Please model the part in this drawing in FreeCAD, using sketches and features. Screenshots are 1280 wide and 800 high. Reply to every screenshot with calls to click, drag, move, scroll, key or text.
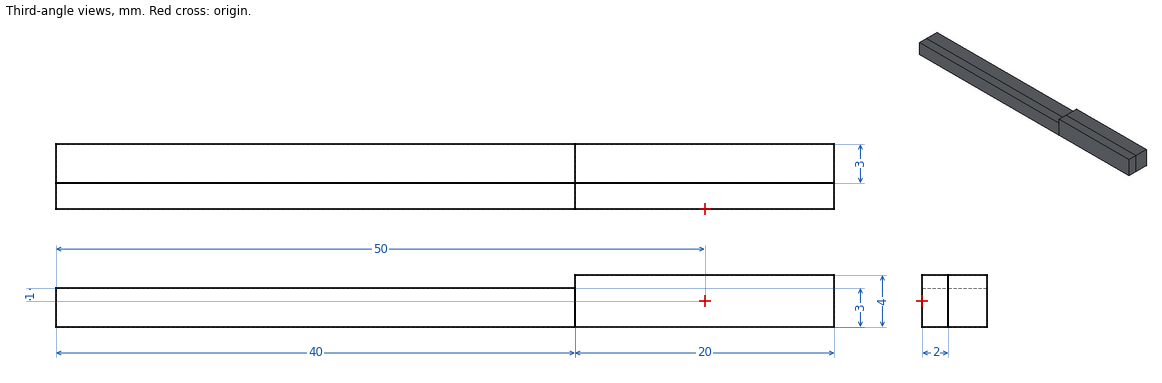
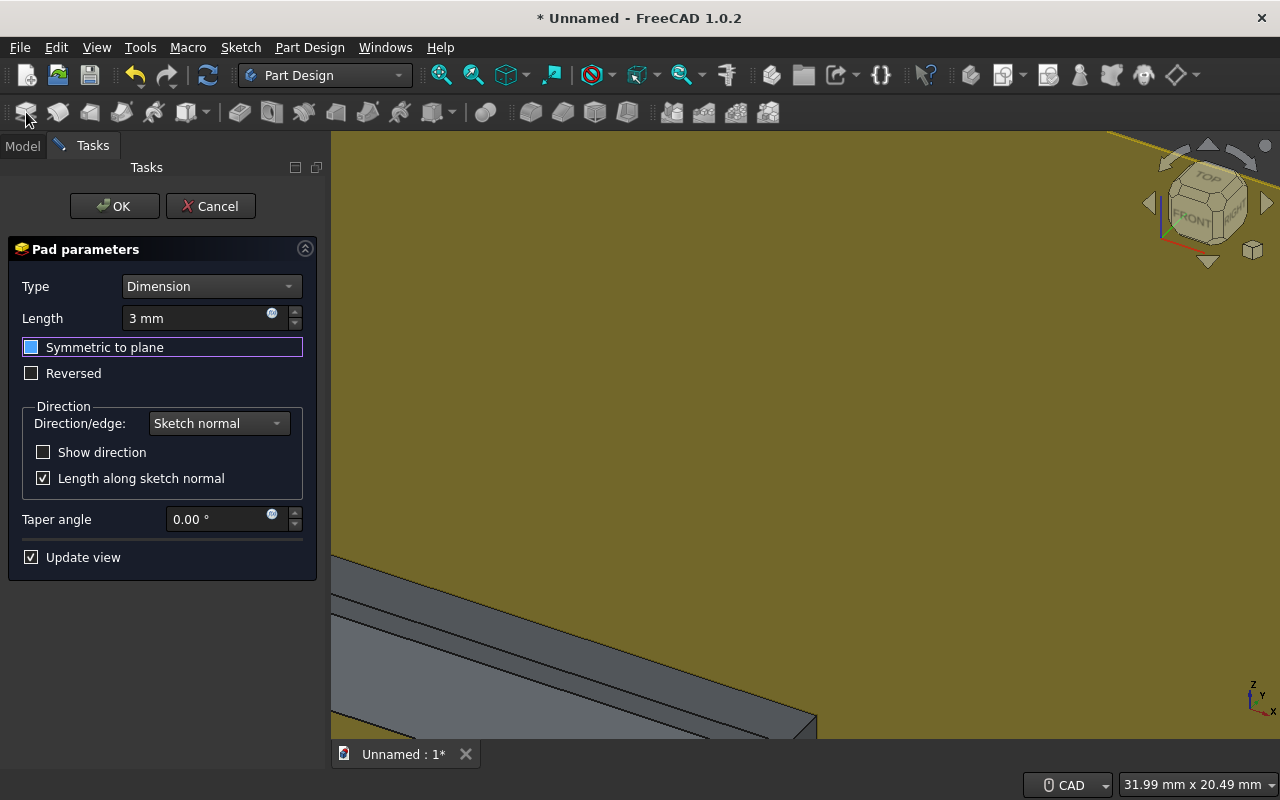
click(30, 373)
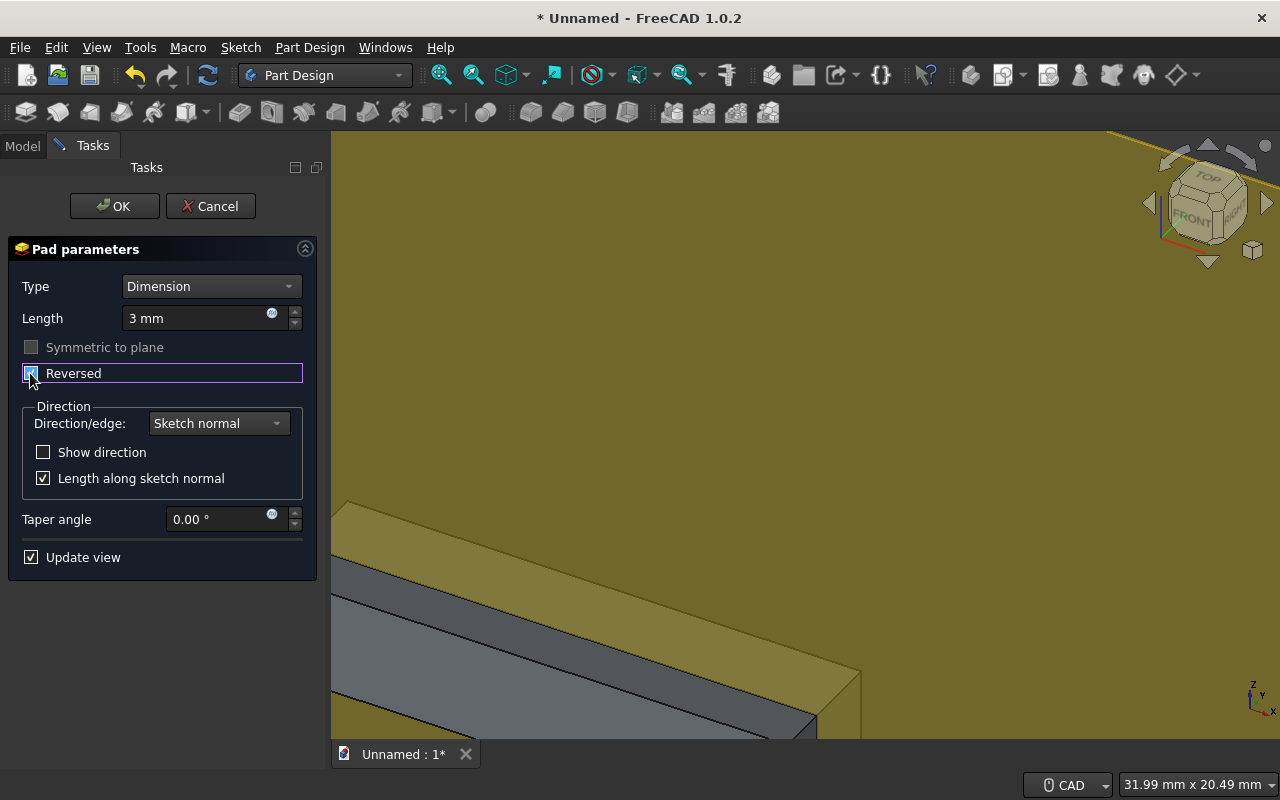
click(115, 206)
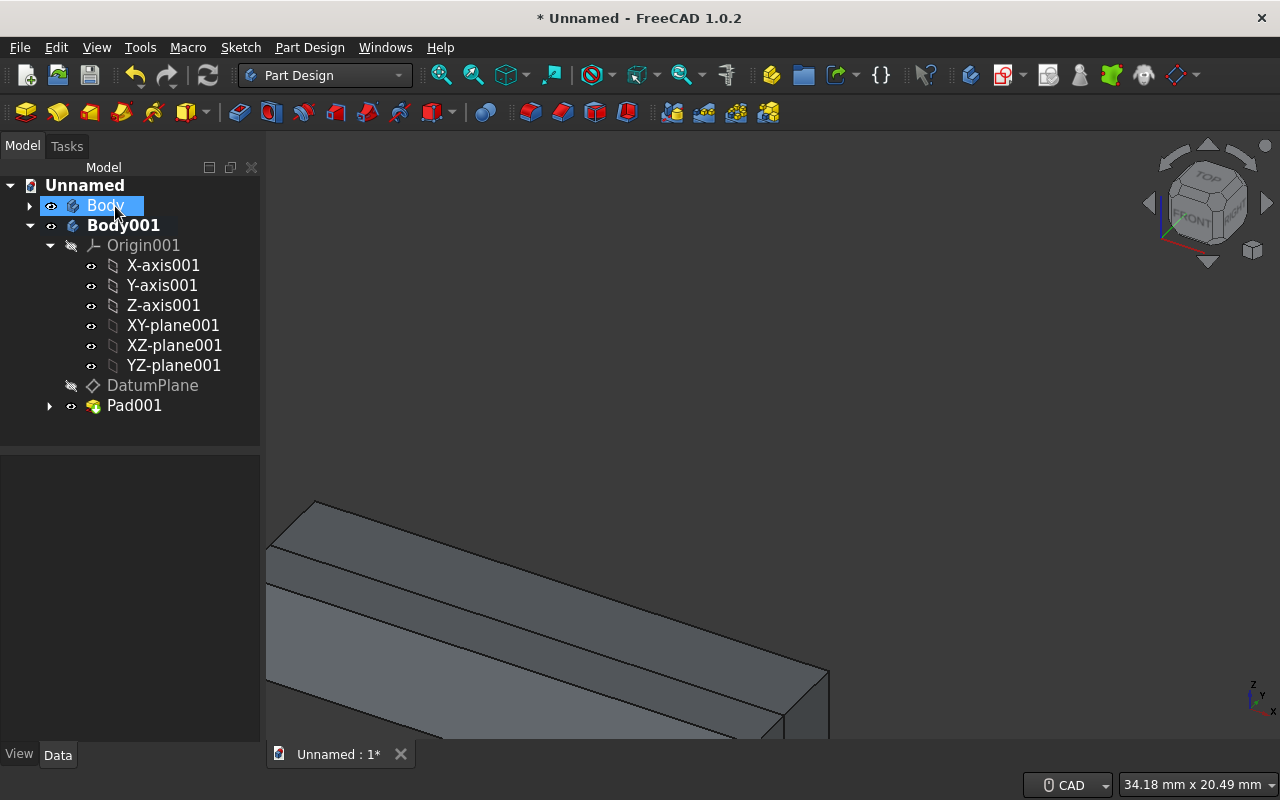
key(v)
key(f)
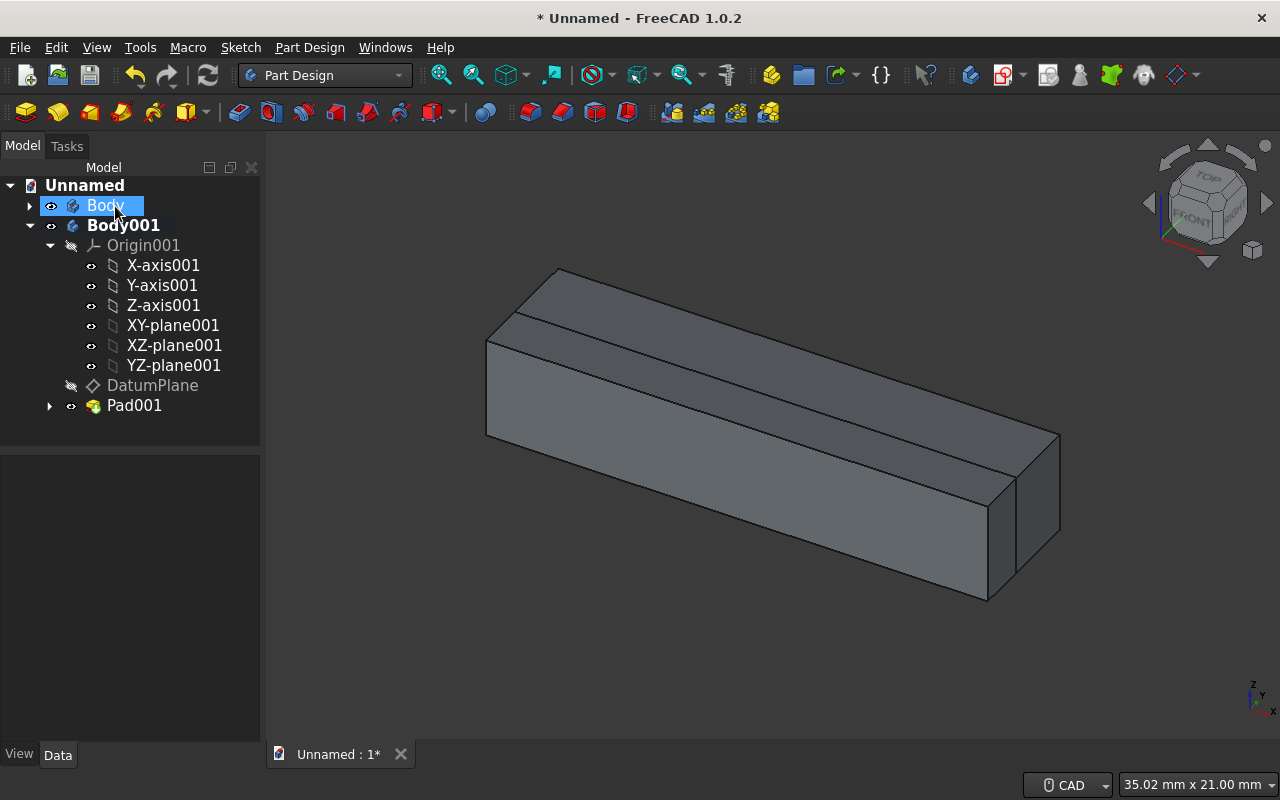
click(972, 76)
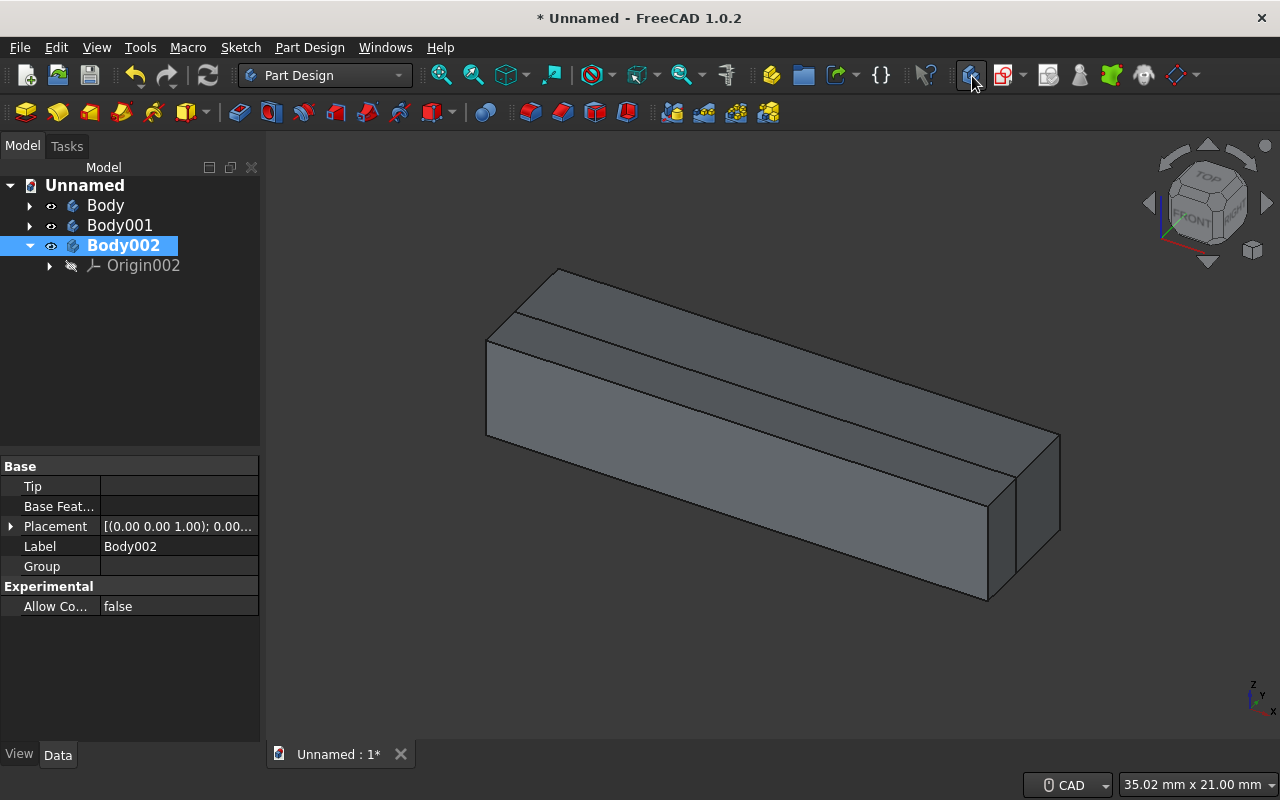
click(306, 699)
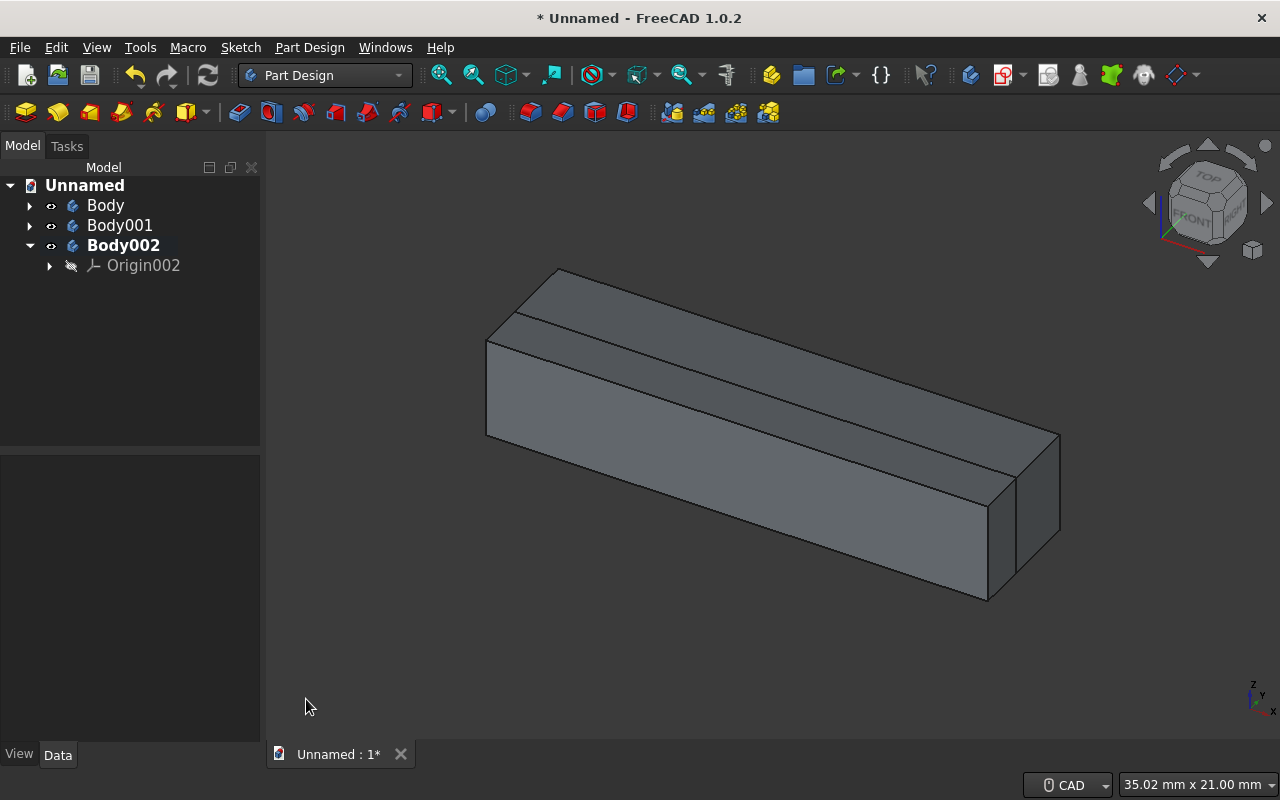
click(1004, 76)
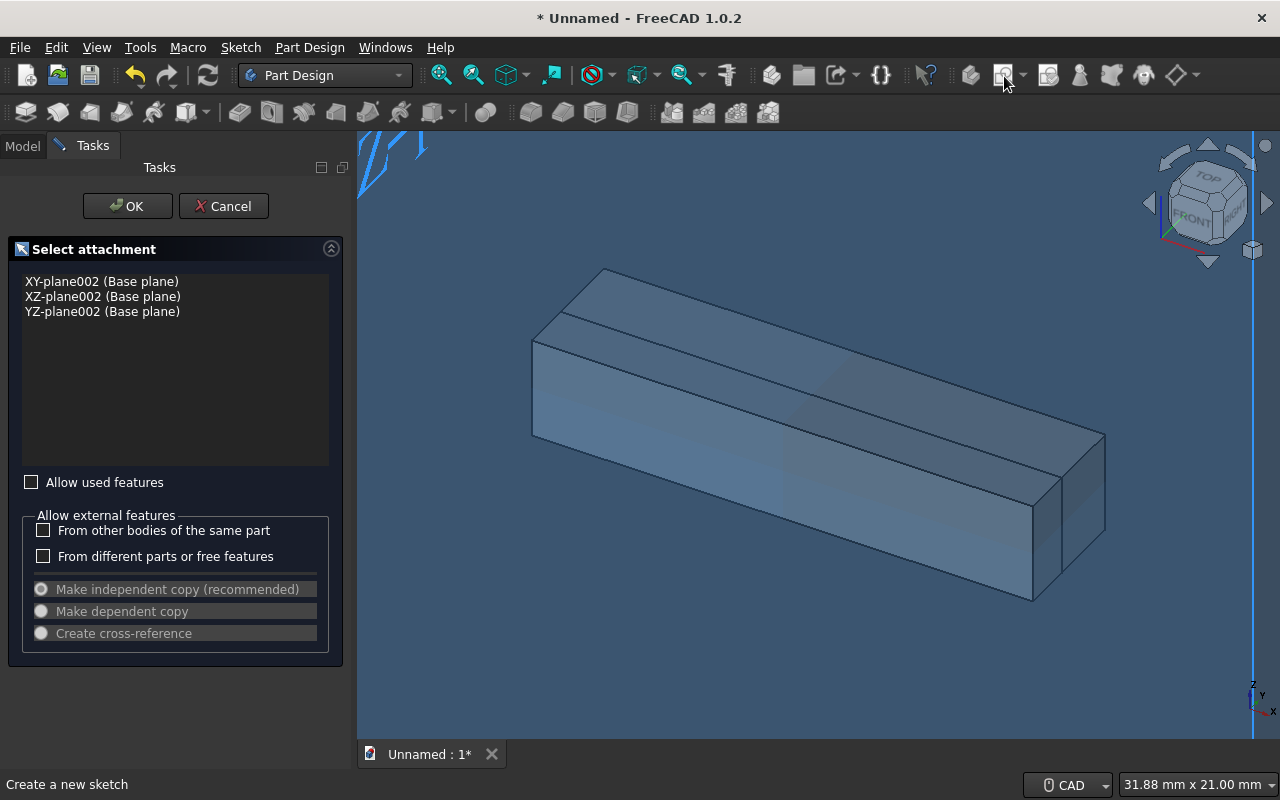
click(82, 296)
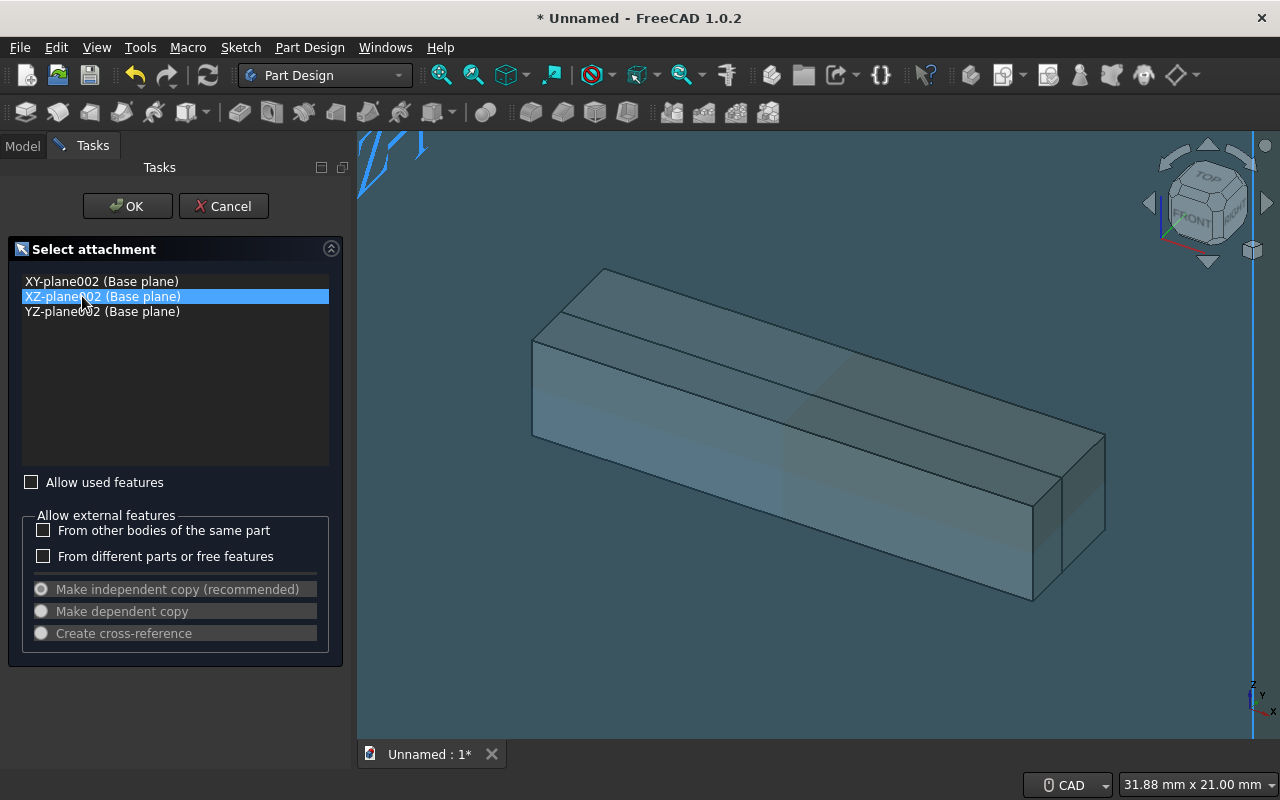
click(128, 206)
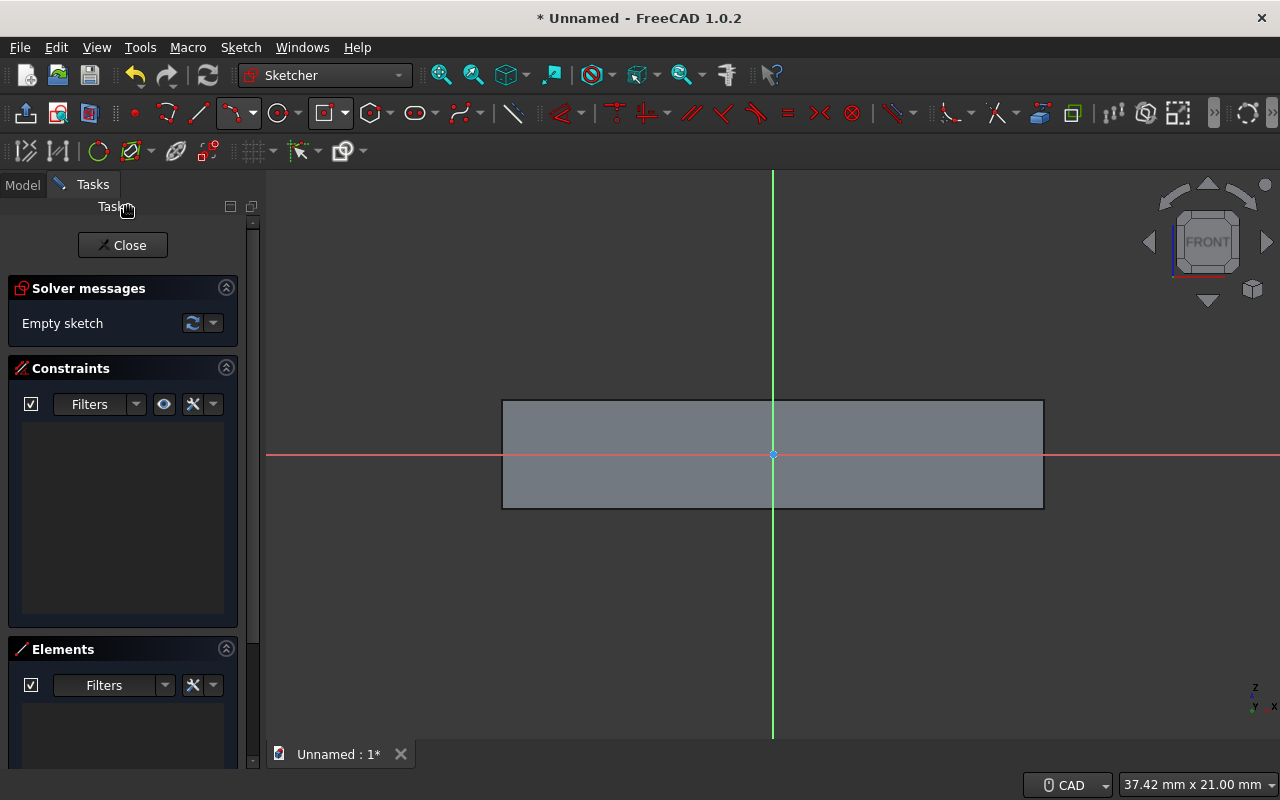
scroll(1115, 443, down, 4)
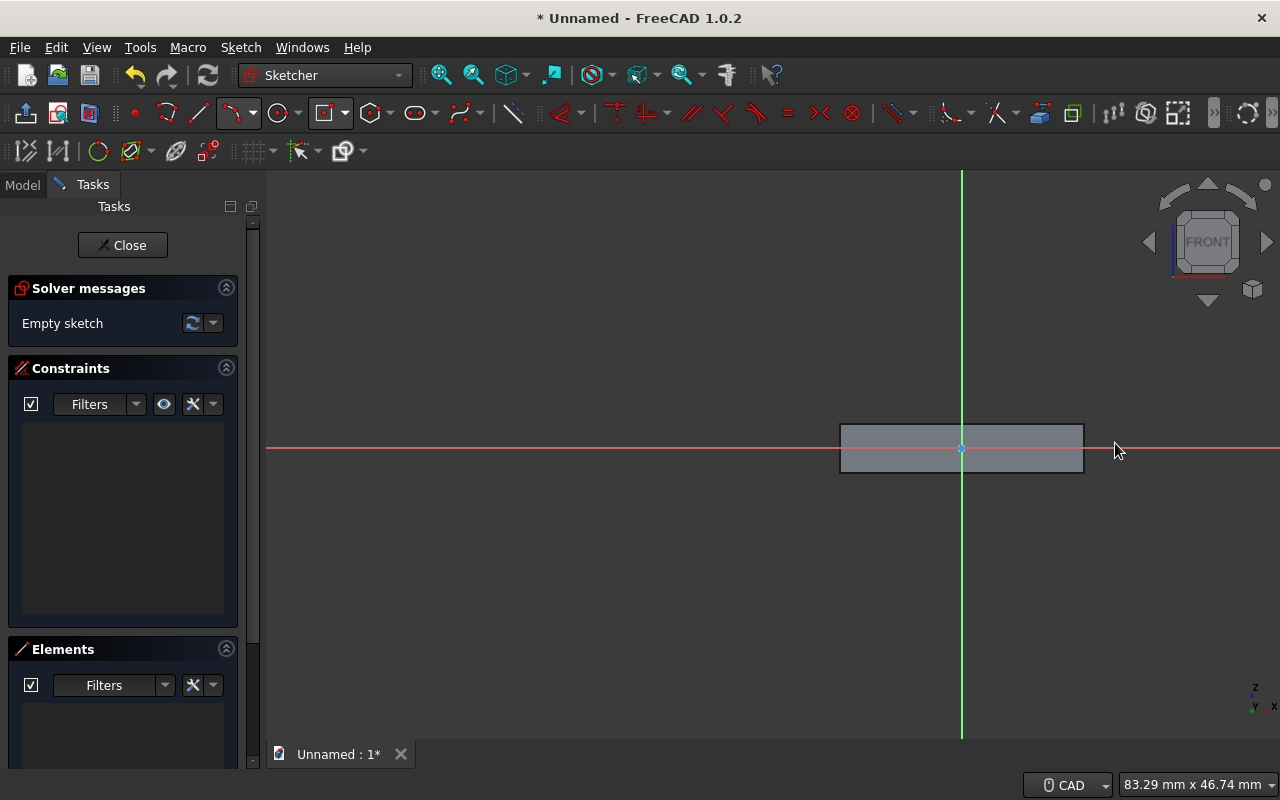
key(g)
key(r)